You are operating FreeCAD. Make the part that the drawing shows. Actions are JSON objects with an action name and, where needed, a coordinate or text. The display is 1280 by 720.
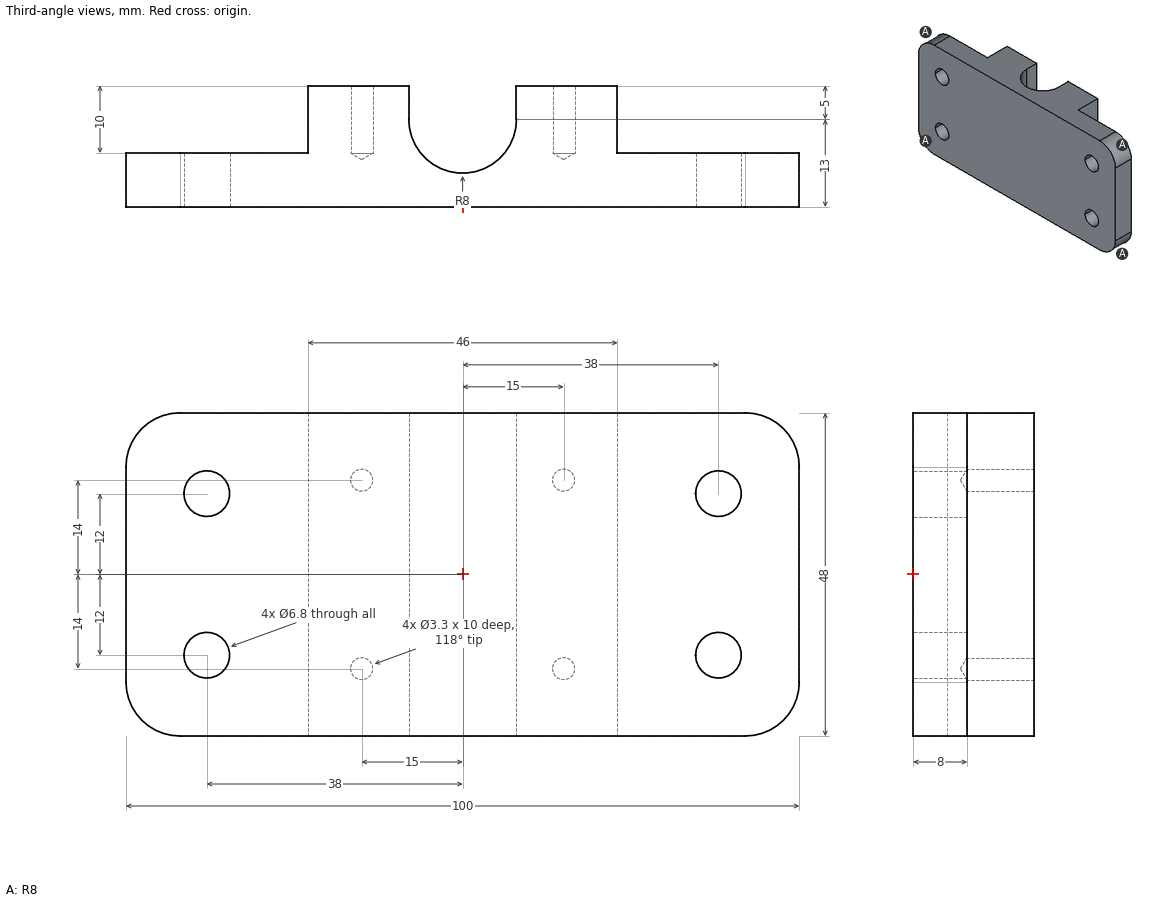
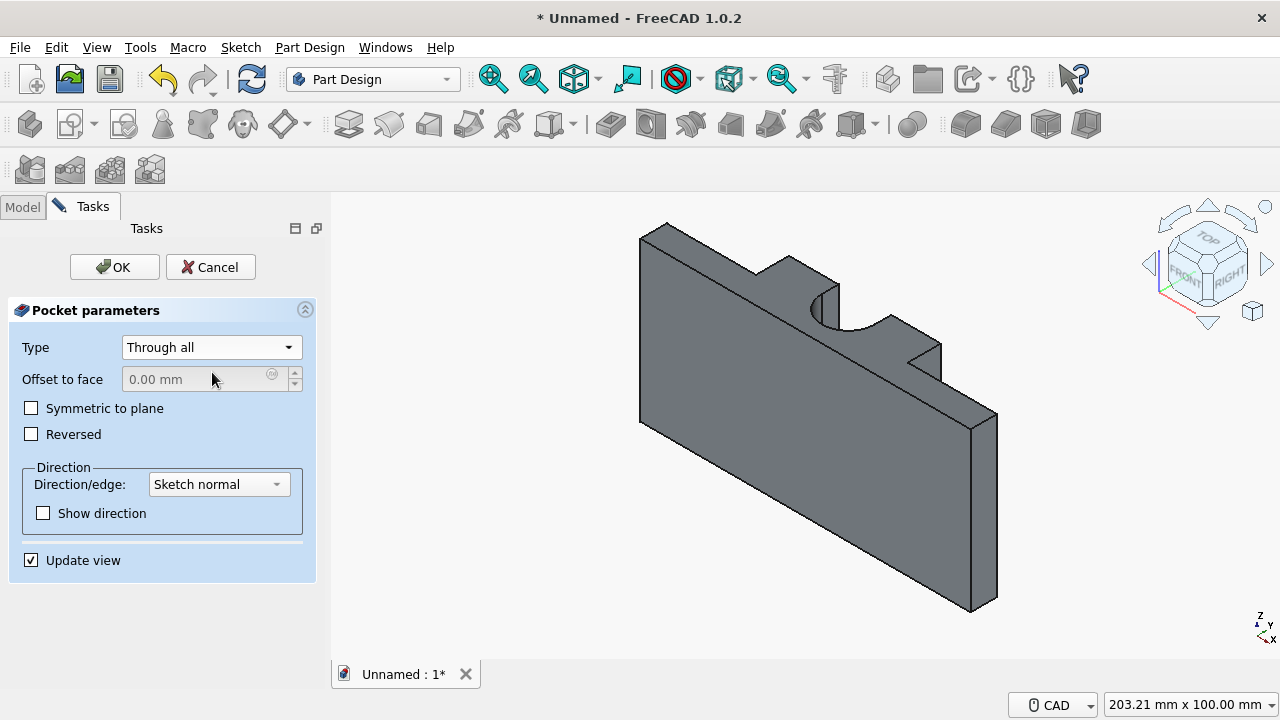
{"action": "left_click", "coordinate": [115, 267]}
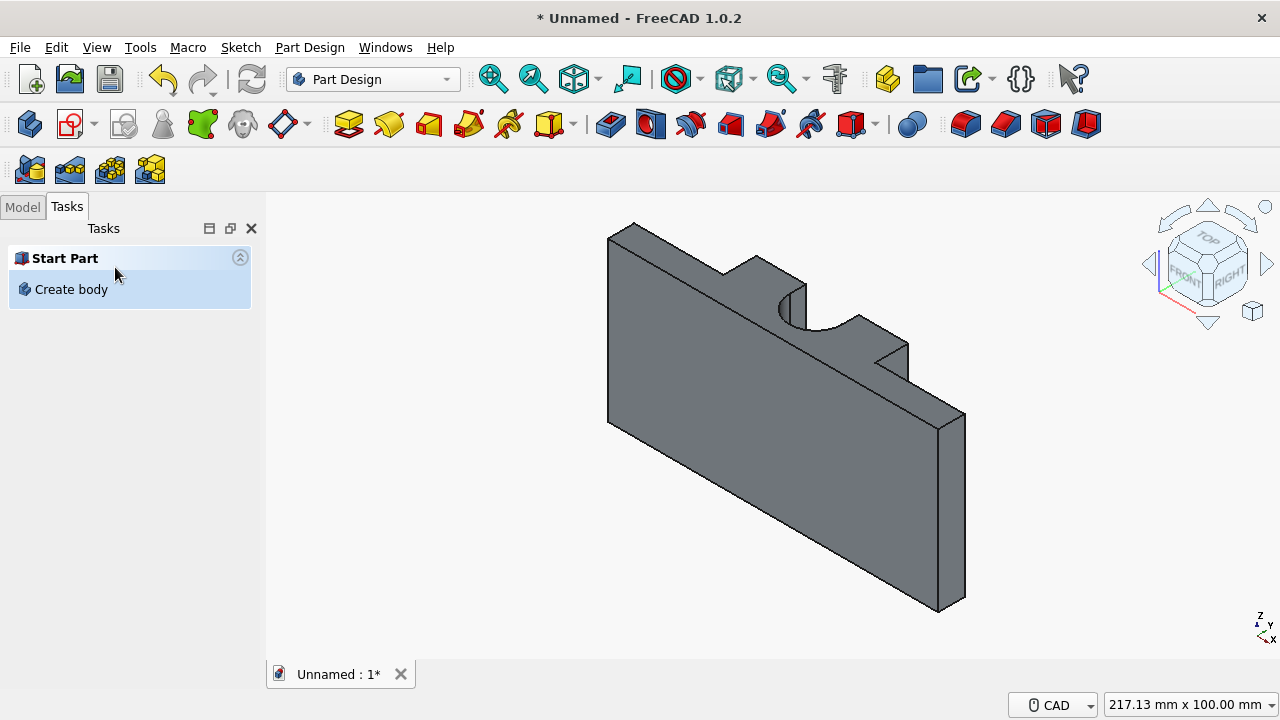
{"action": "left_click", "coordinate": [951, 421]}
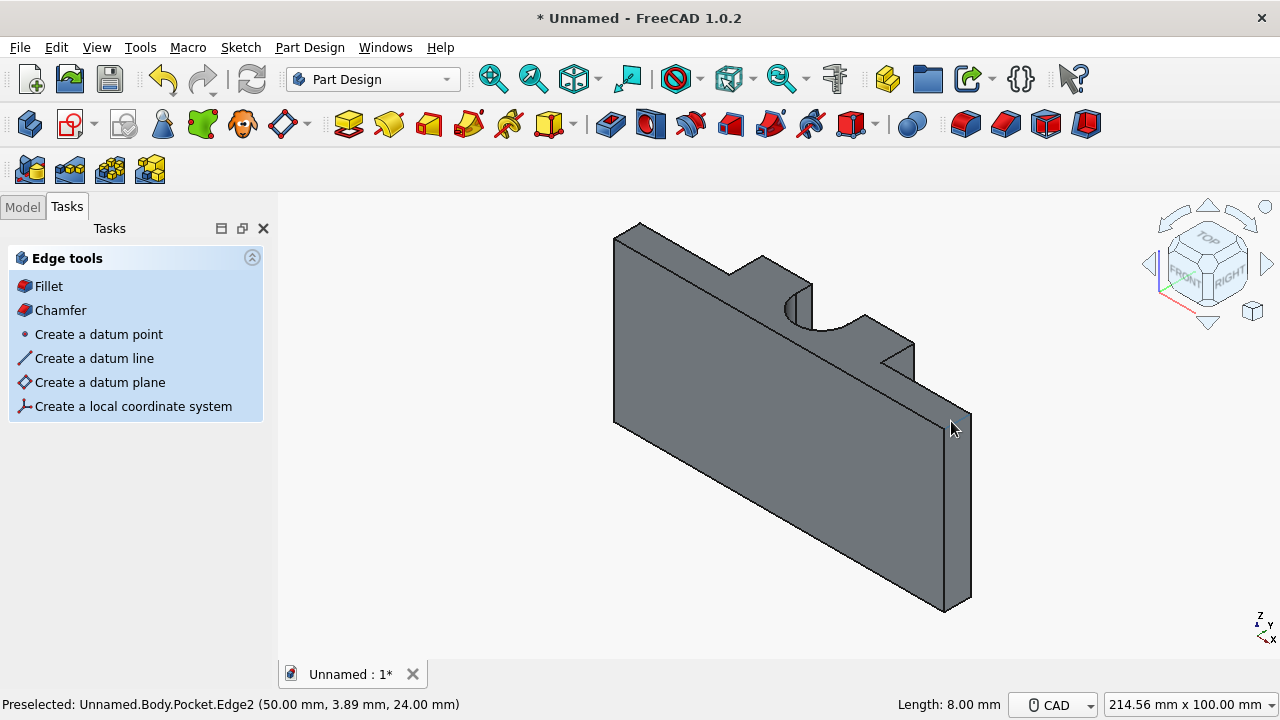
{"action": "key", "text": "2"}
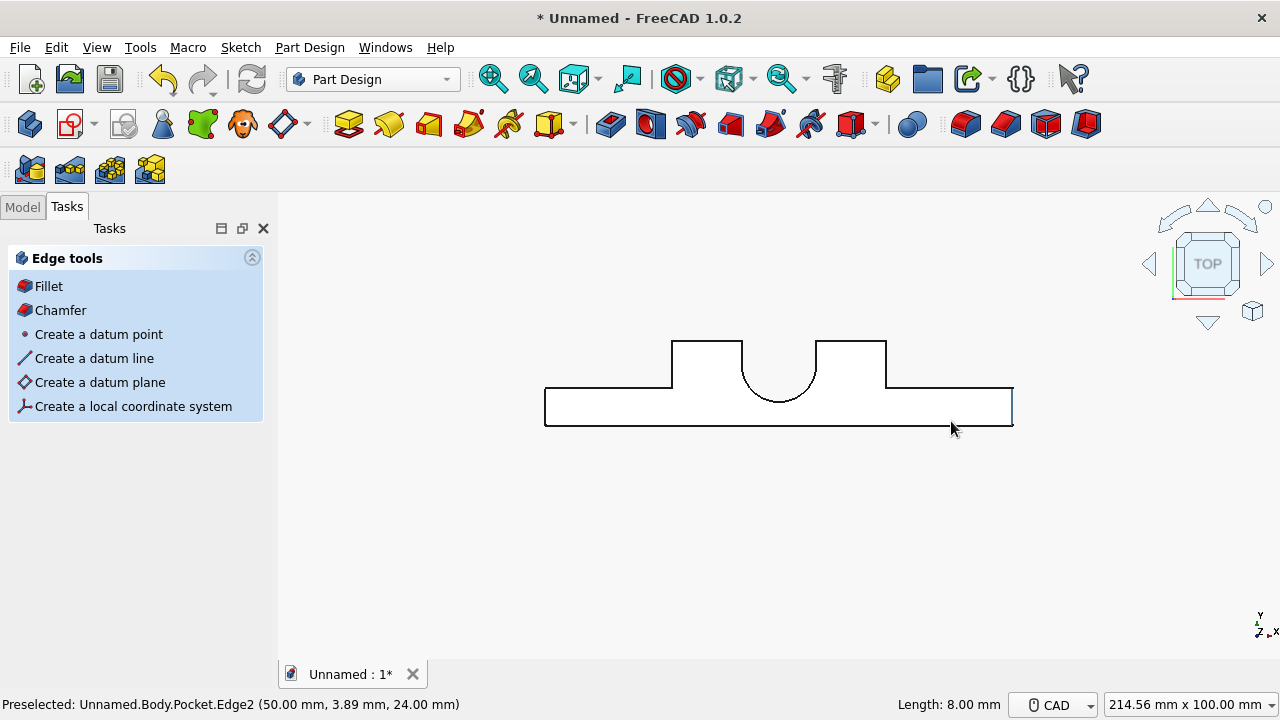
{"action": "left_click", "coordinate": [545, 406], "text": "ctrl"}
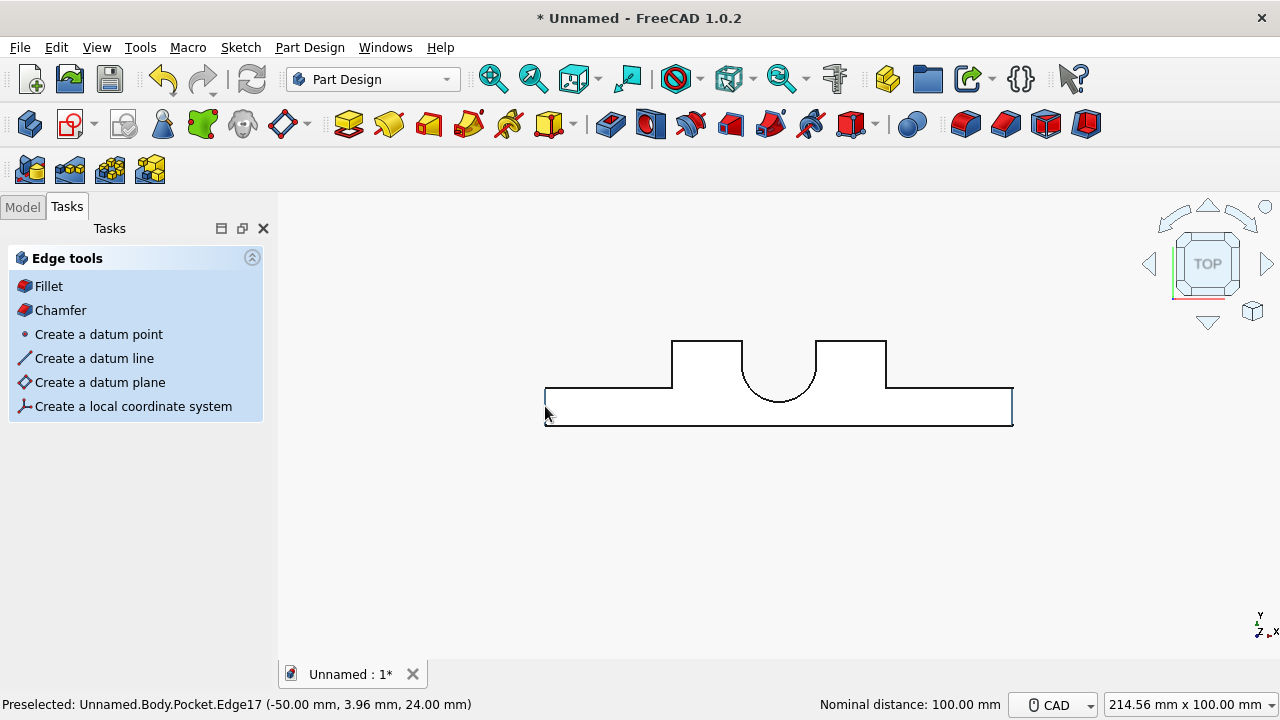
{"action": "key", "text": "0"}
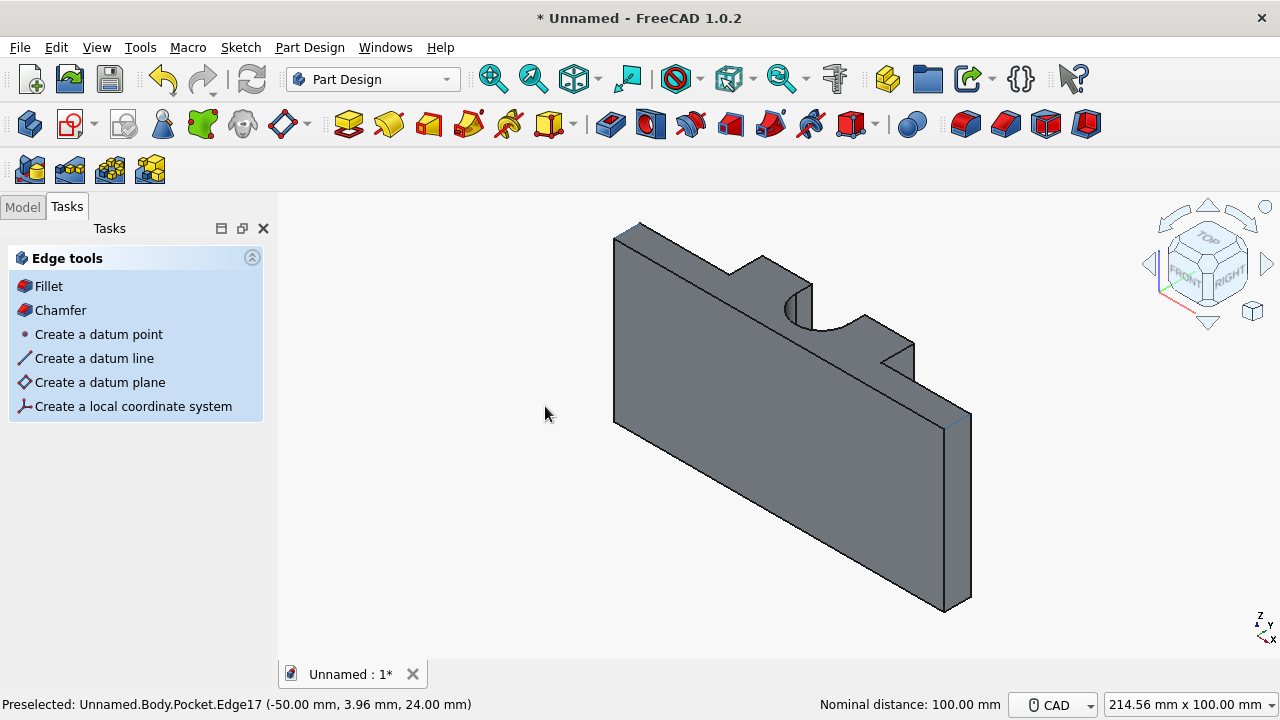
{"action": "key", "text": "1"}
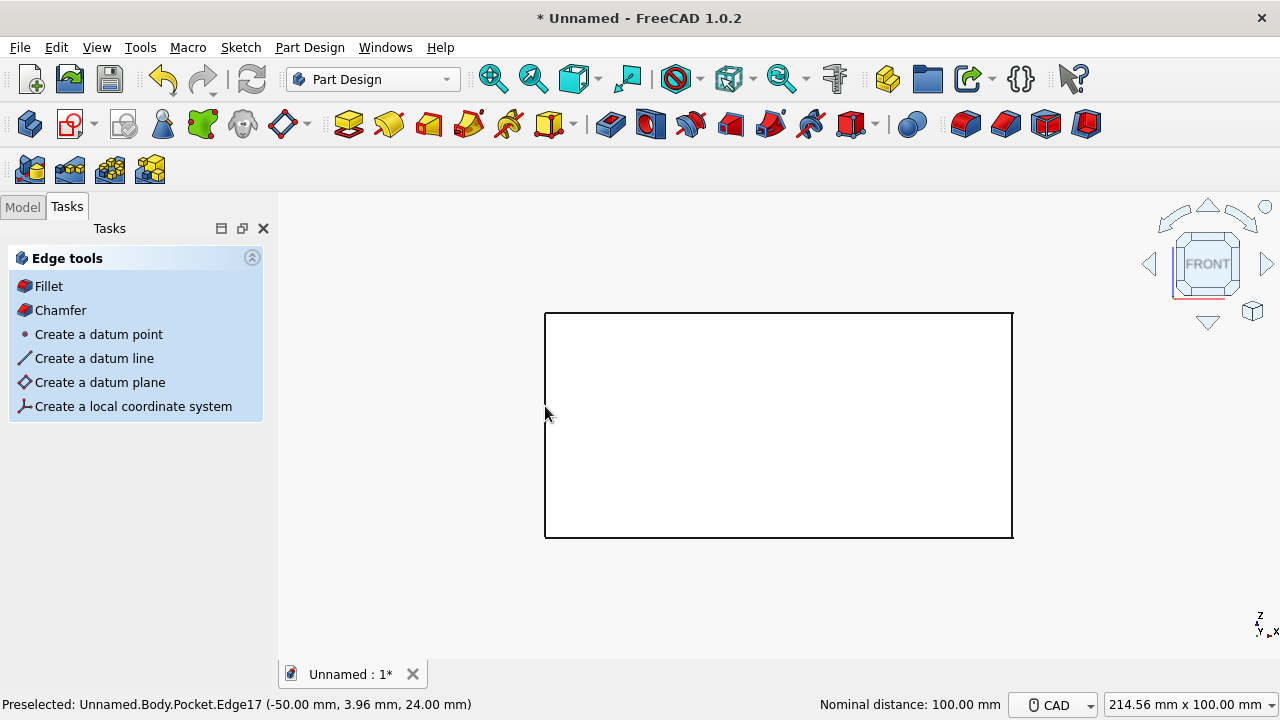
{"action": "key", "text": "3"}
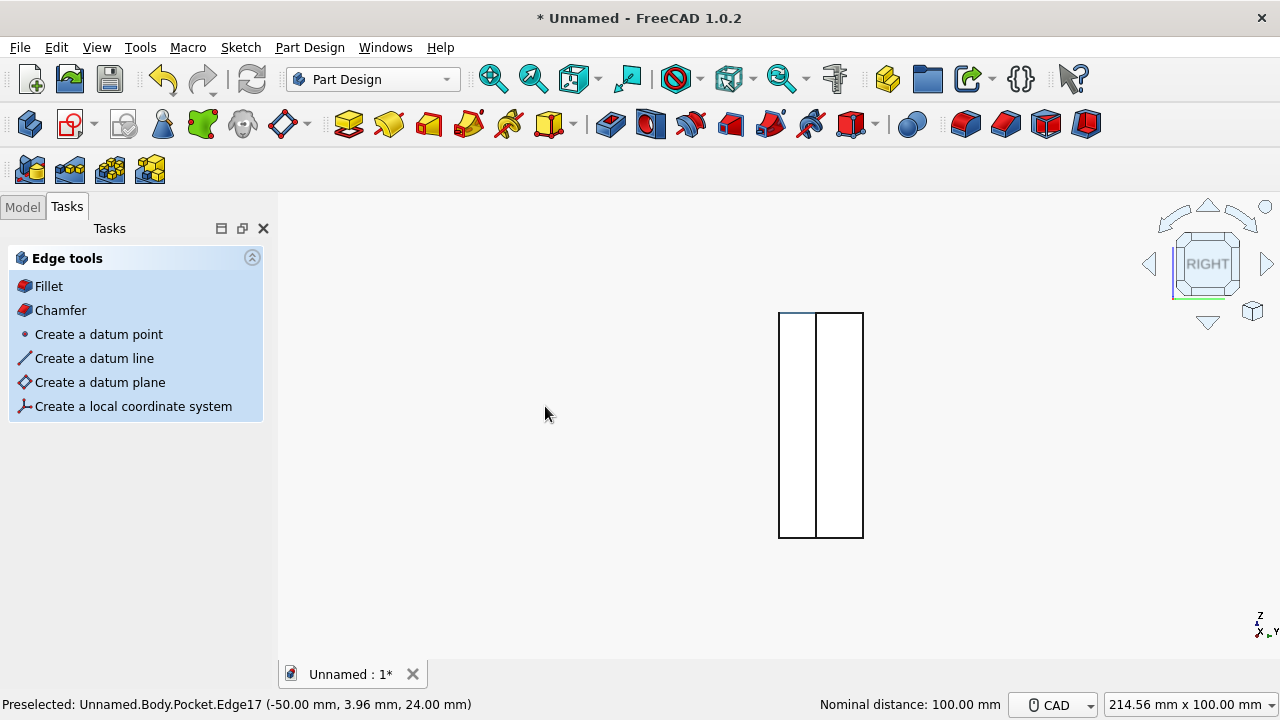
{"action": "left_click", "coordinate": [798, 537], "text": "ctrl"}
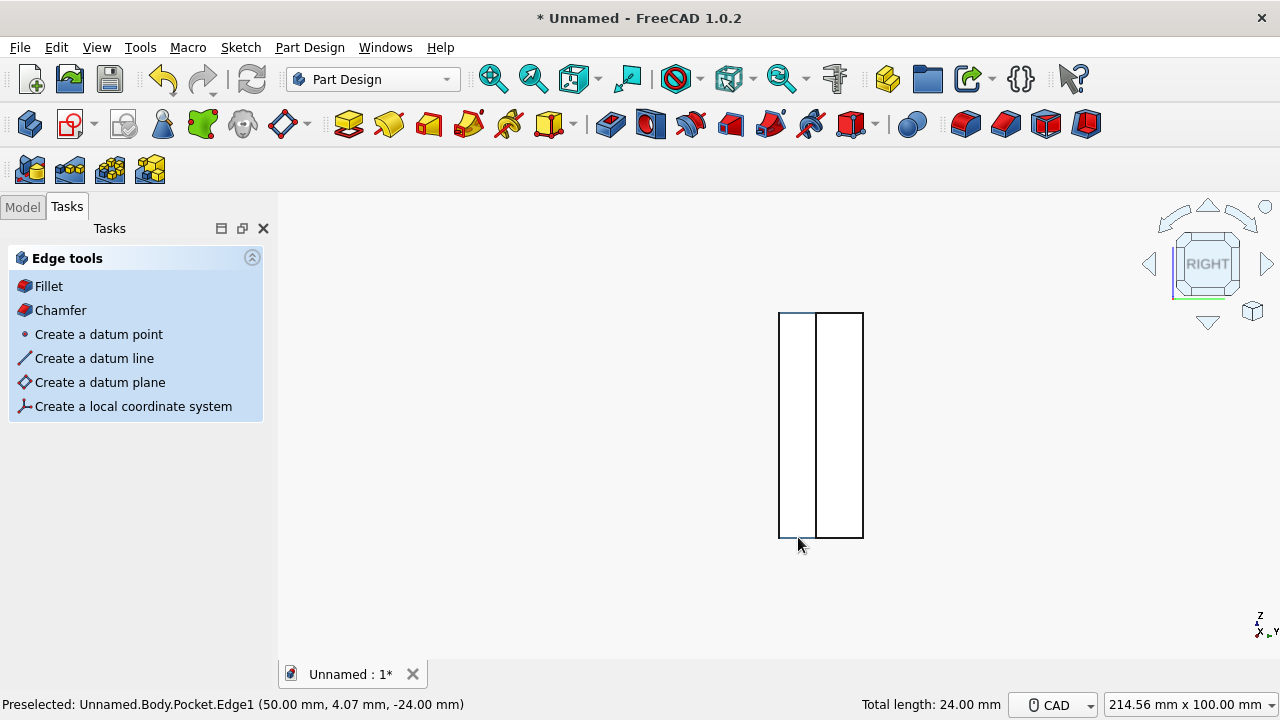
{"action": "key", "text": "5"}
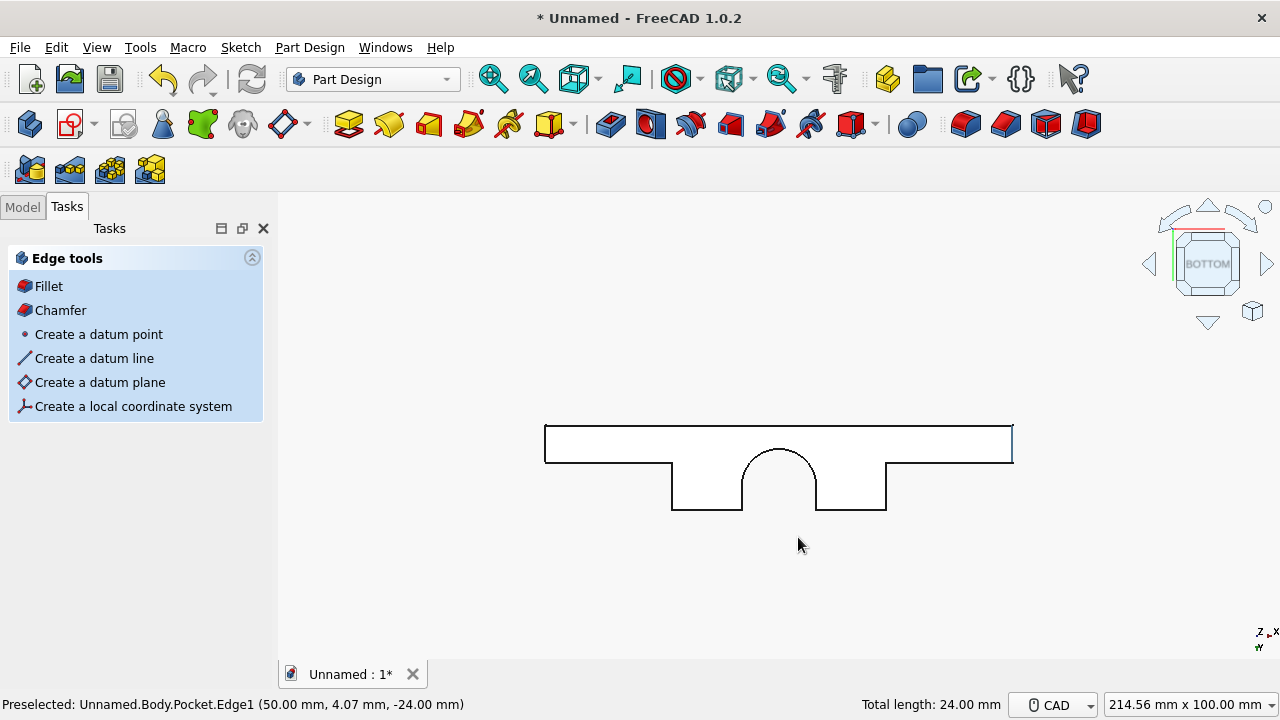
{"action": "left_click", "coordinate": [545, 443], "text": "ctrl"}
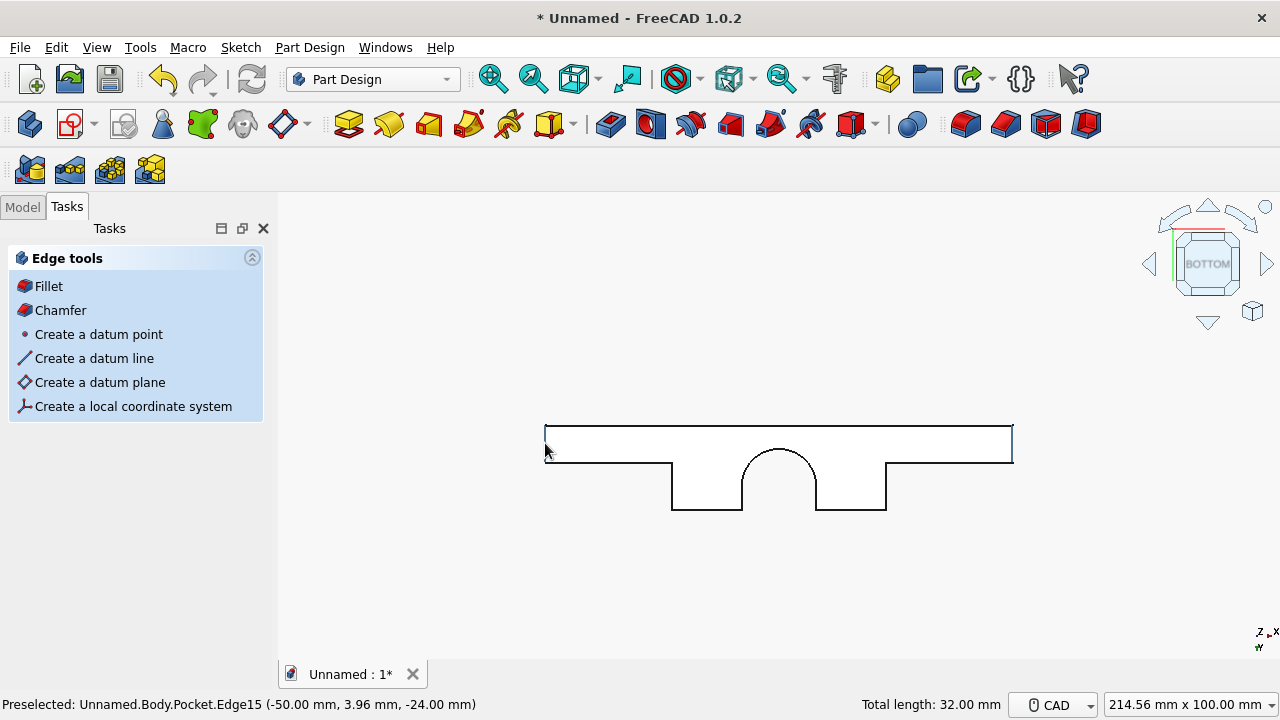
{"action": "left_click", "coordinate": [966, 124]}